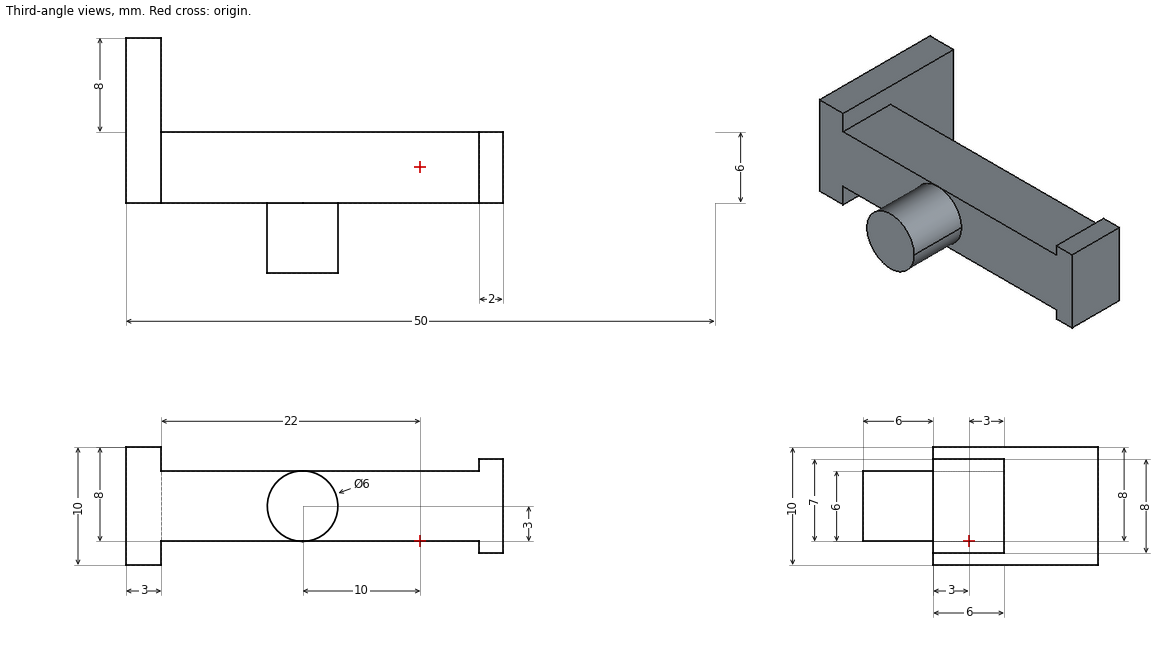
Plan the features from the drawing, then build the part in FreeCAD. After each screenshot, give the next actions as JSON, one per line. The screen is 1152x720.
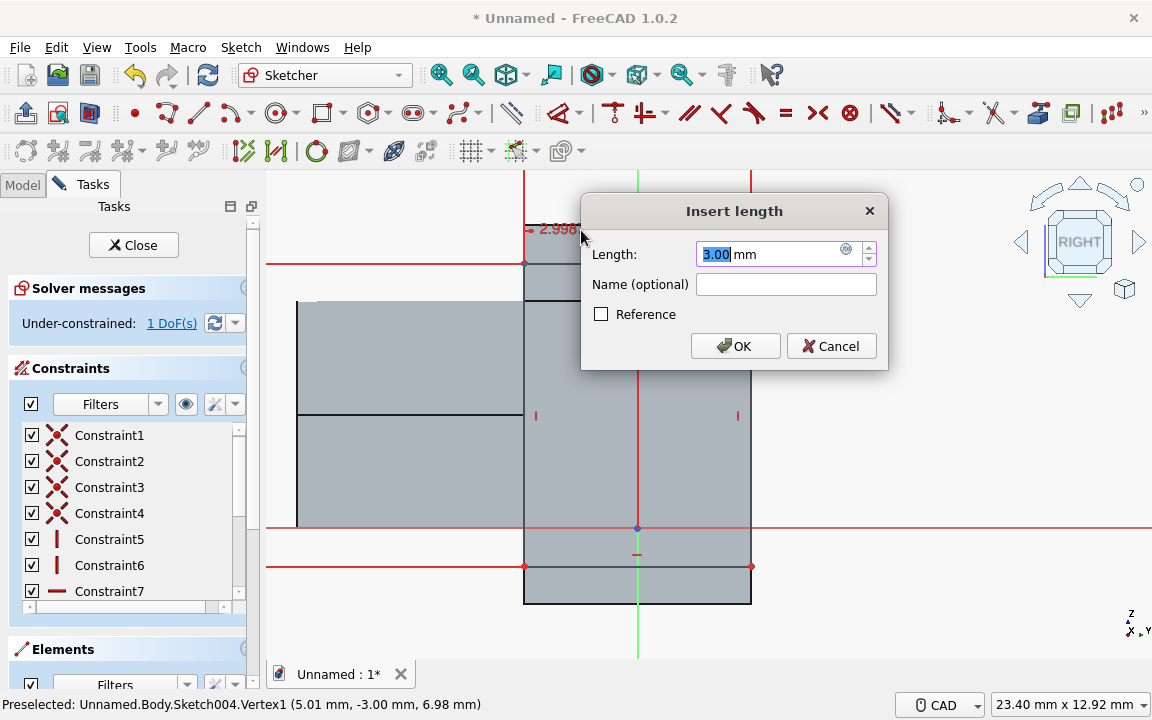
{"action": "type", "text": "3"}
{"action": "key", "text": "Return"}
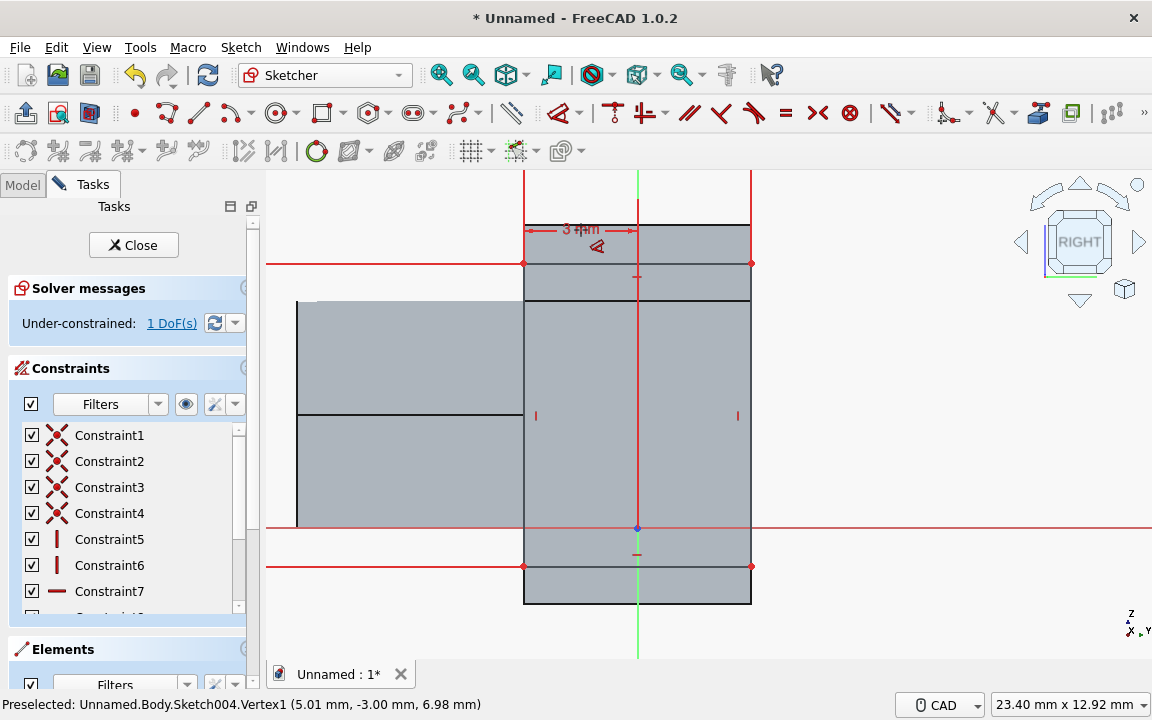
{"action": "left_click", "coordinate": [524, 264]}
{"action": "left_click", "coordinate": [490, 396]}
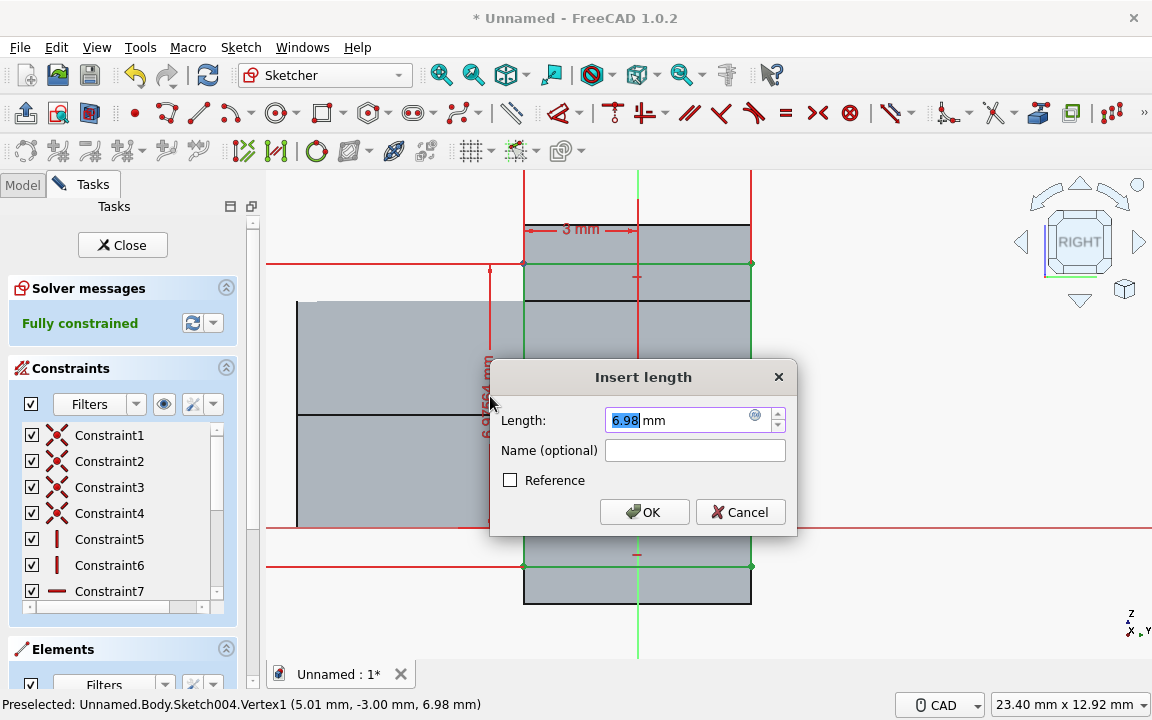
{"action": "type", "text": "7"}
{"action": "key", "text": "Return"}
{"action": "key", "text": "Escape"}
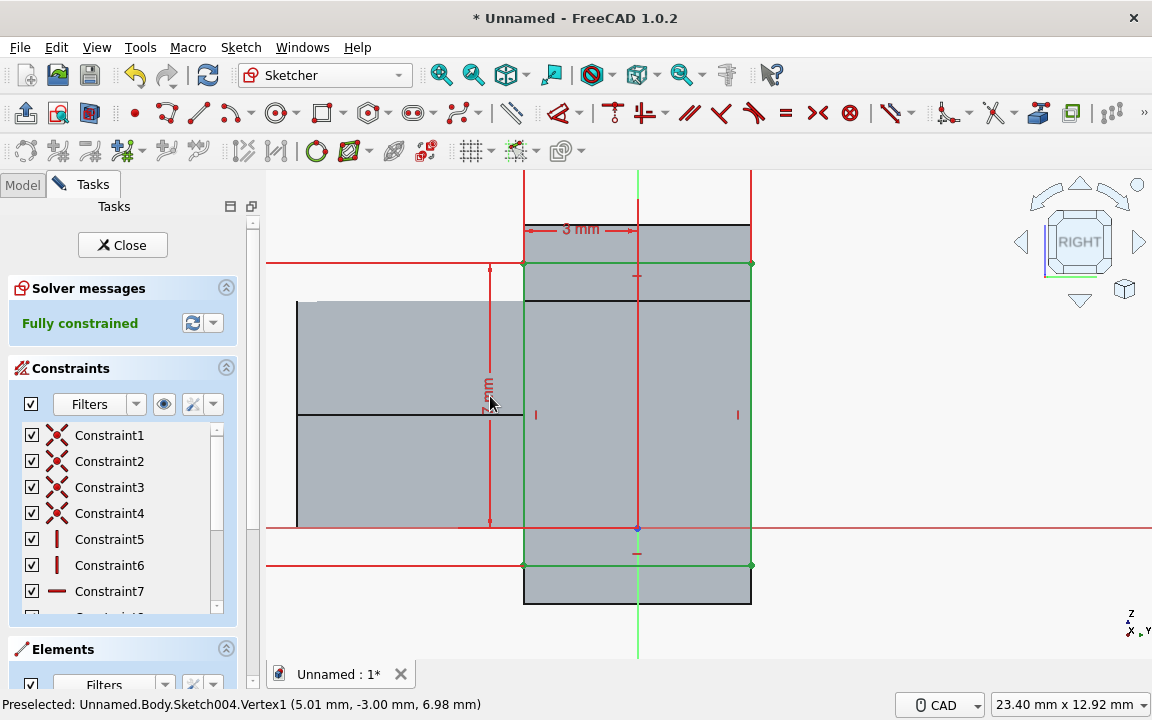
{"action": "left_click", "coordinate": [123, 245]}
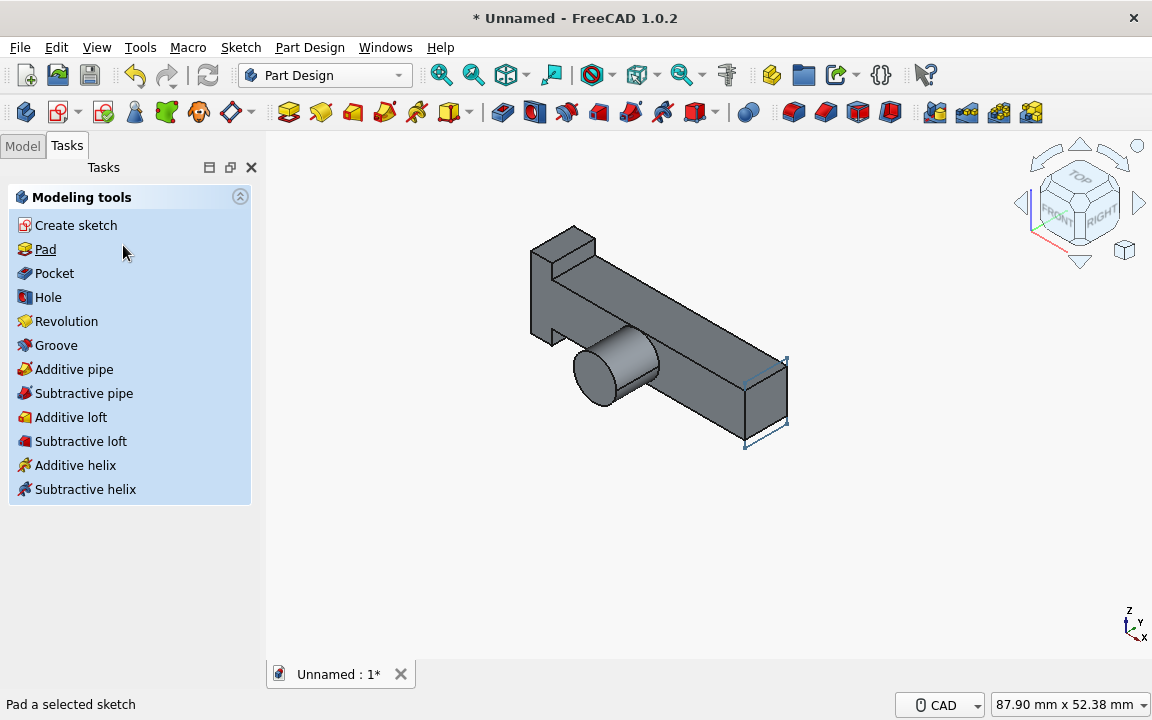
{"action": "left_click", "coordinate": [290, 112]}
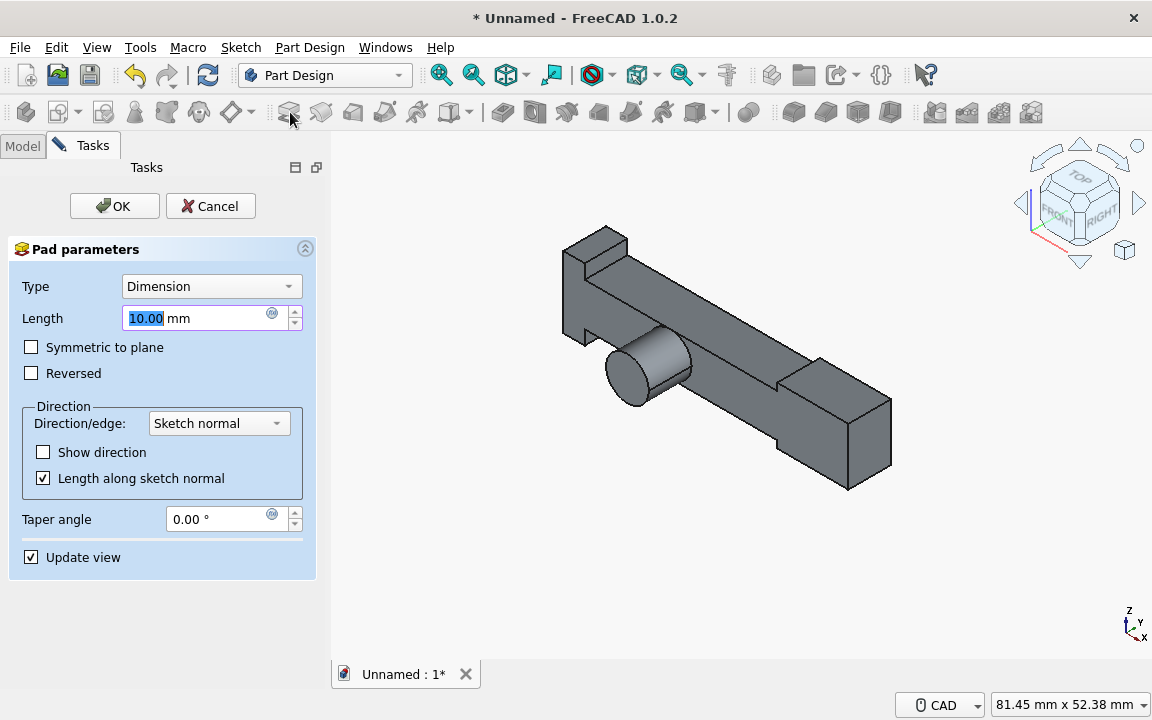
{"action": "type", "text": "2"}
{"action": "key", "text": "Tab"}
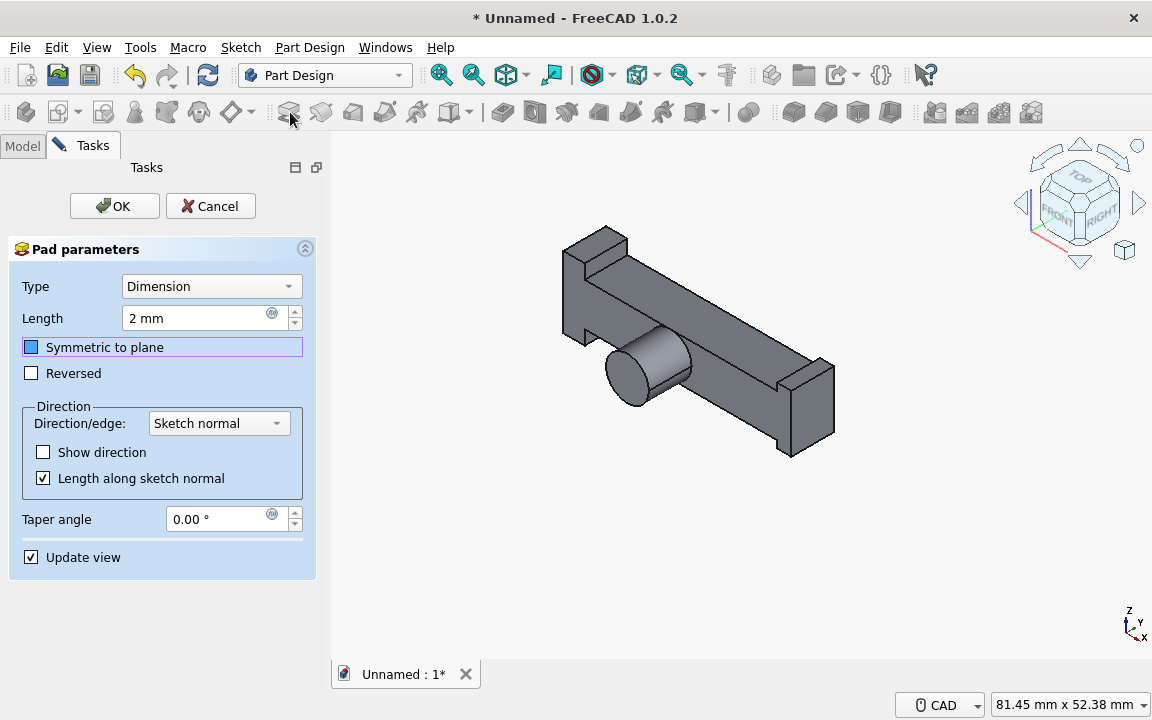
{"action": "left_click", "coordinate": [115, 206]}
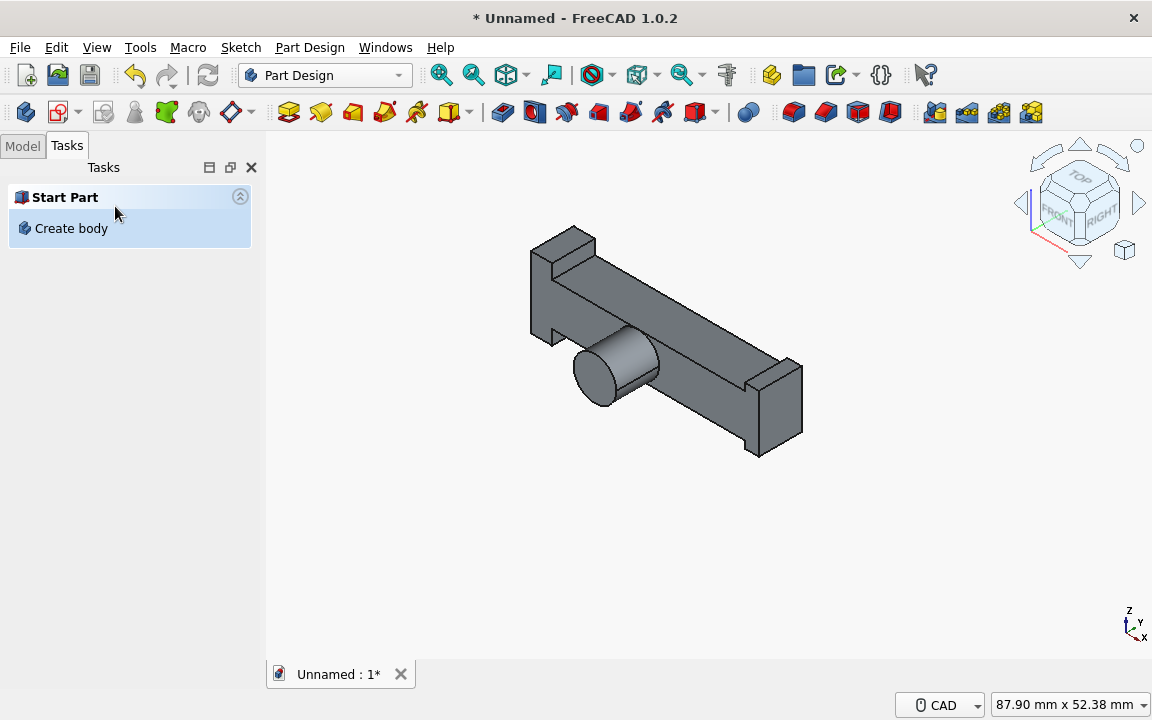
{"action": "key", "text": "4"}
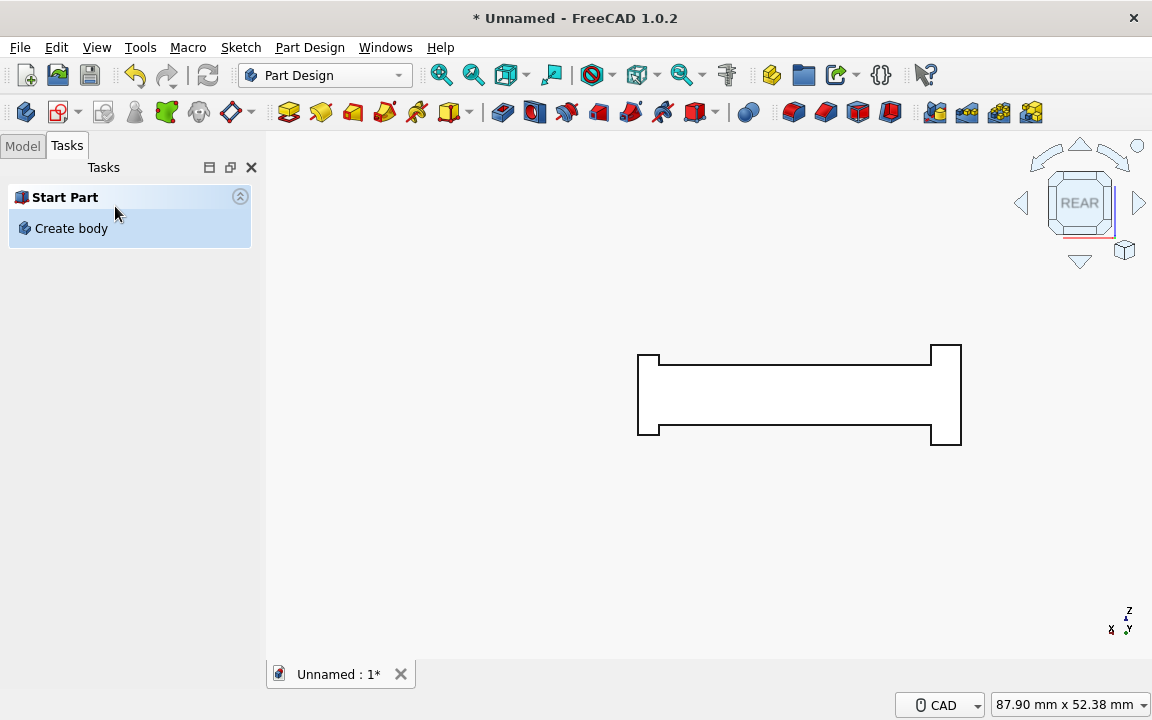
{"action": "left_click", "coordinate": [442, 76]}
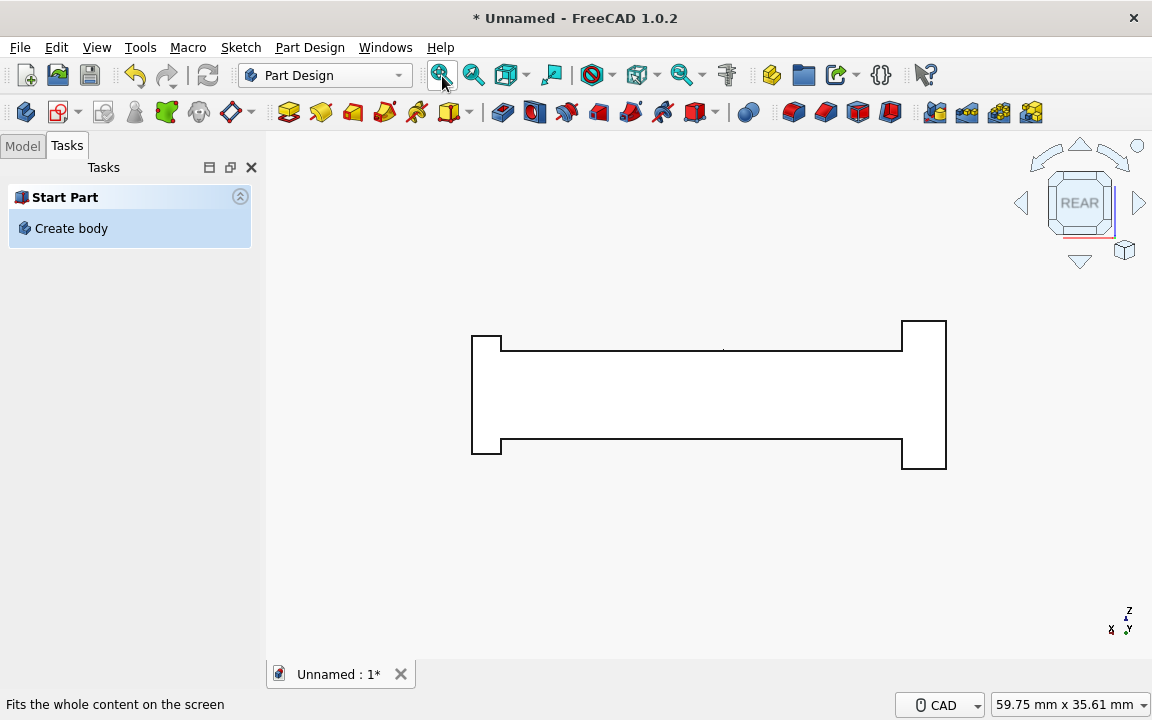
{"action": "left_click", "coordinate": [573, 394]}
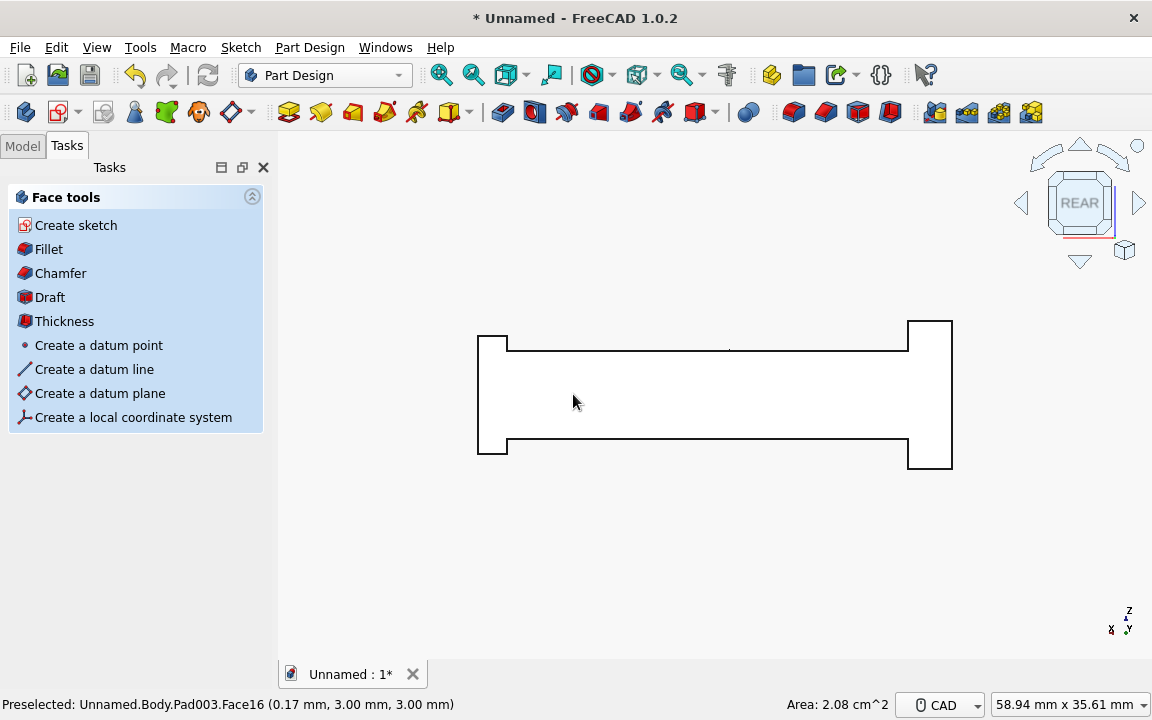
{"action": "left_click", "coordinate": [58, 112]}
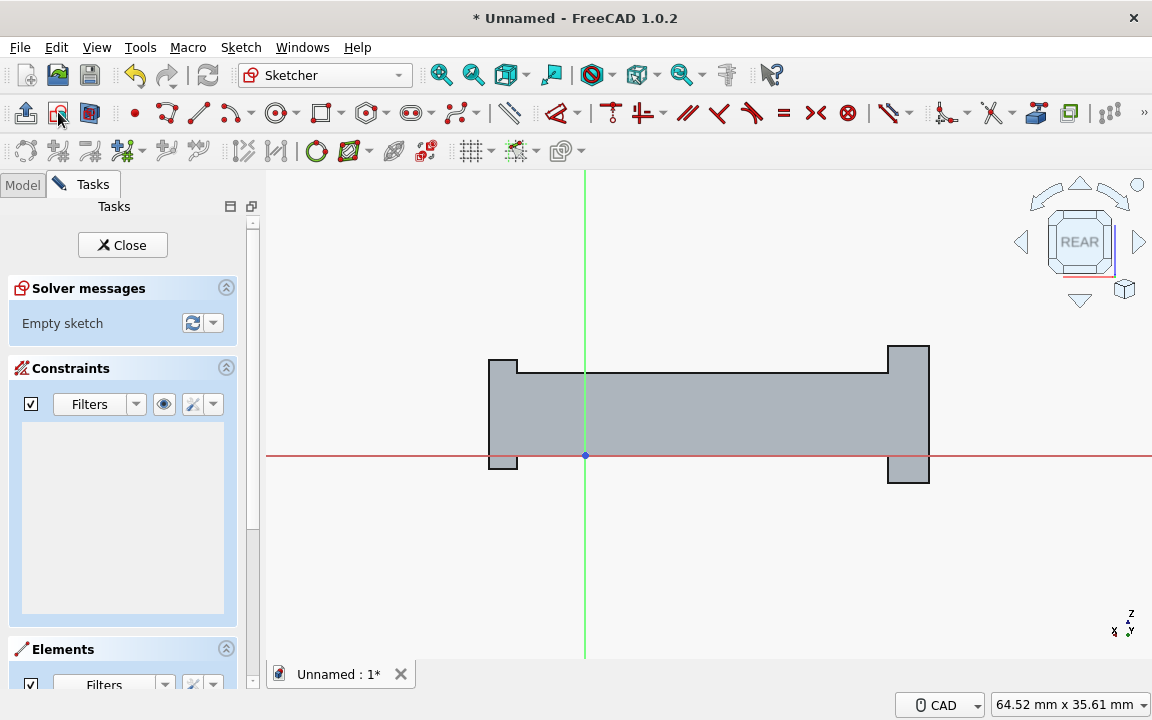
{"action": "scroll", "coordinate": [987, 414], "scroll_direction": "up", "scroll_amount": 4}